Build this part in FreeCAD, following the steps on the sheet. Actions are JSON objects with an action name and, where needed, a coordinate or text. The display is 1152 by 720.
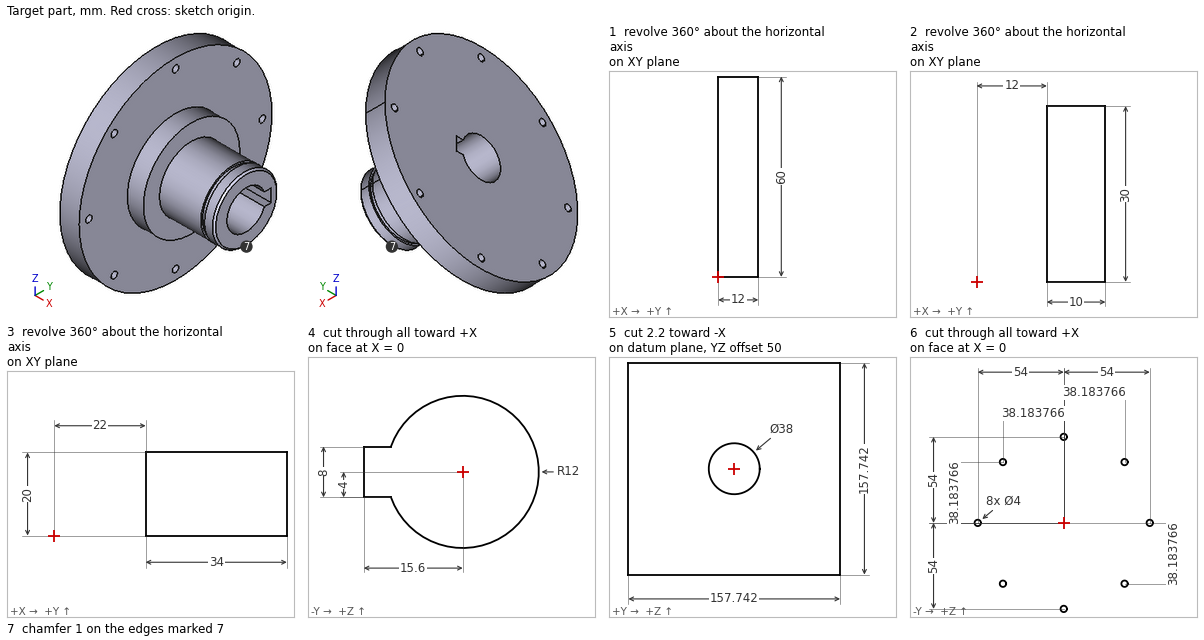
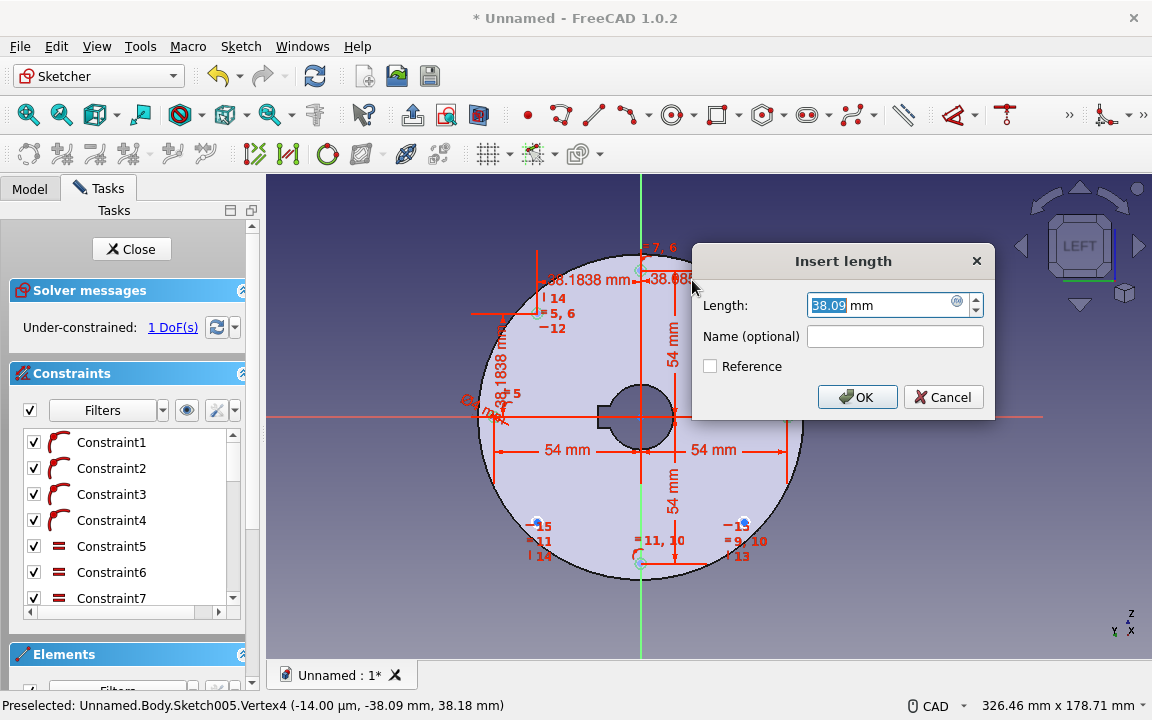
{"action": "type", "text": "38.183766"}
{"action": "key", "text": "Return"}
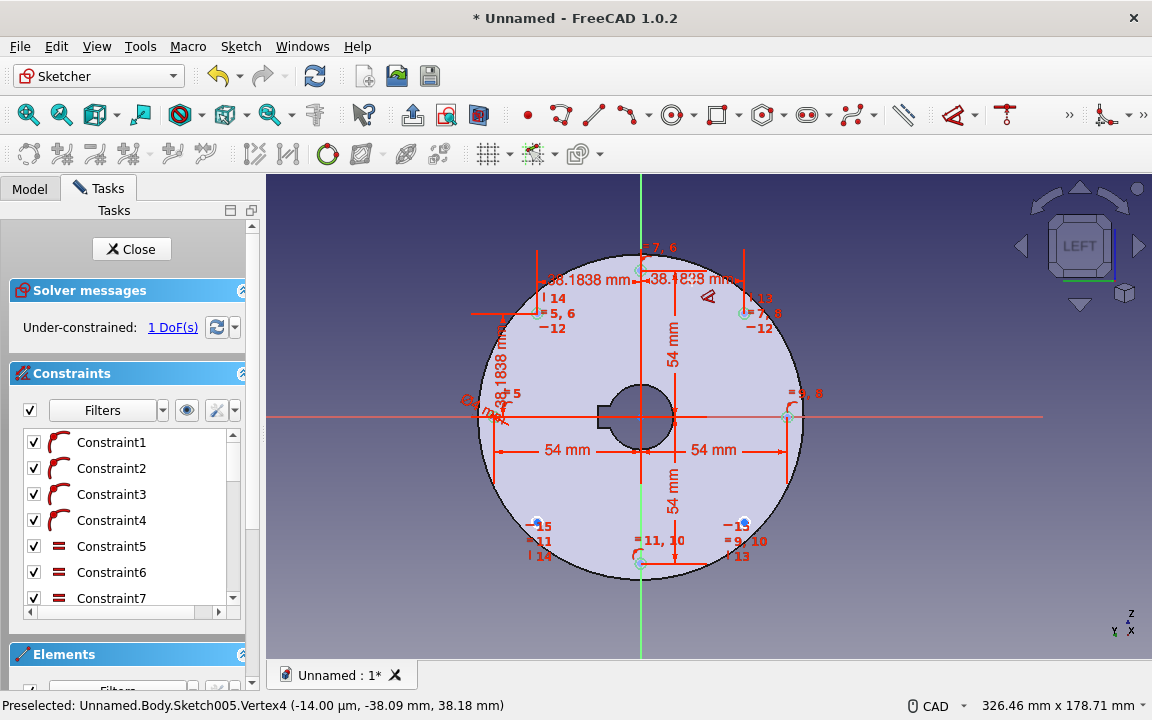
{"action": "left_click", "coordinate": [744, 522]}
{"action": "left_click", "coordinate": [778, 494]}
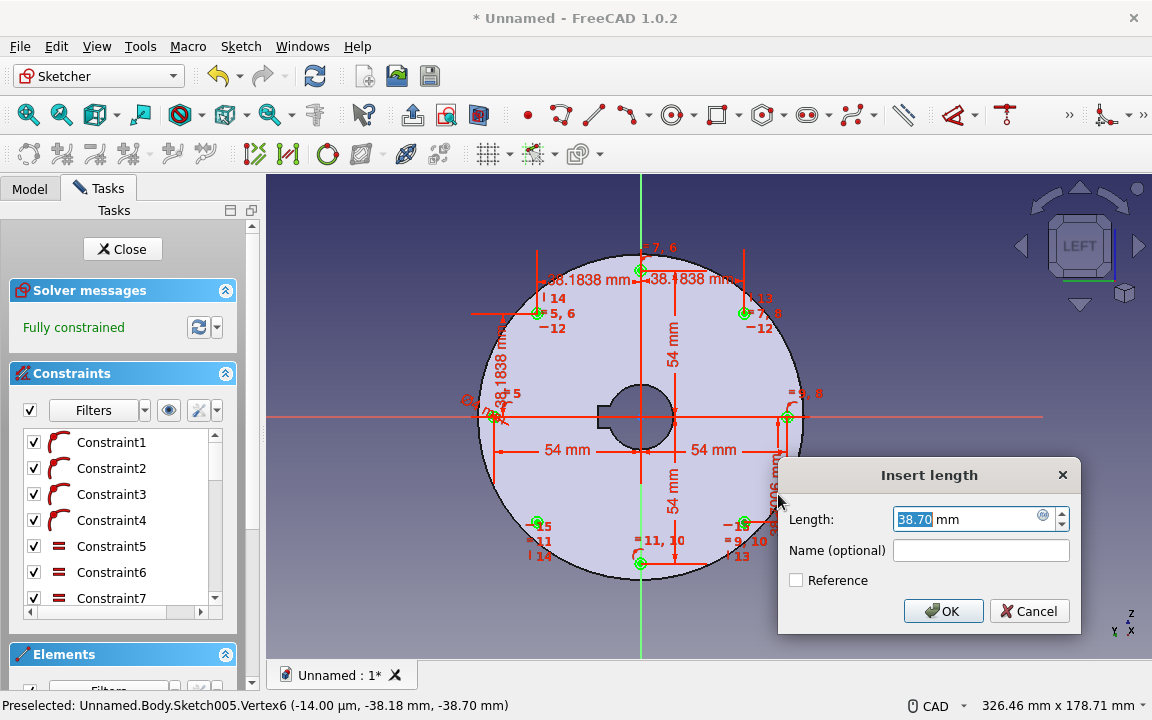
{"action": "type", "text": "38.183766"}
{"action": "key", "text": "Return"}
{"action": "key", "text": "Escape"}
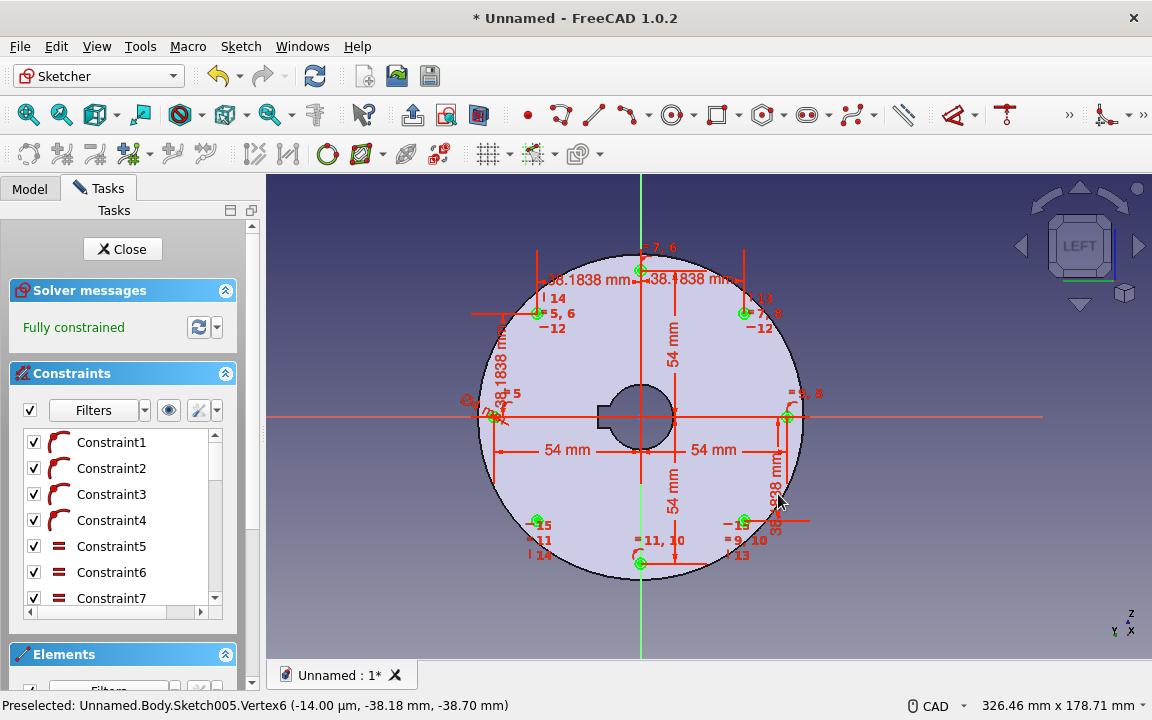
{"action": "left_click", "coordinate": [123, 249]}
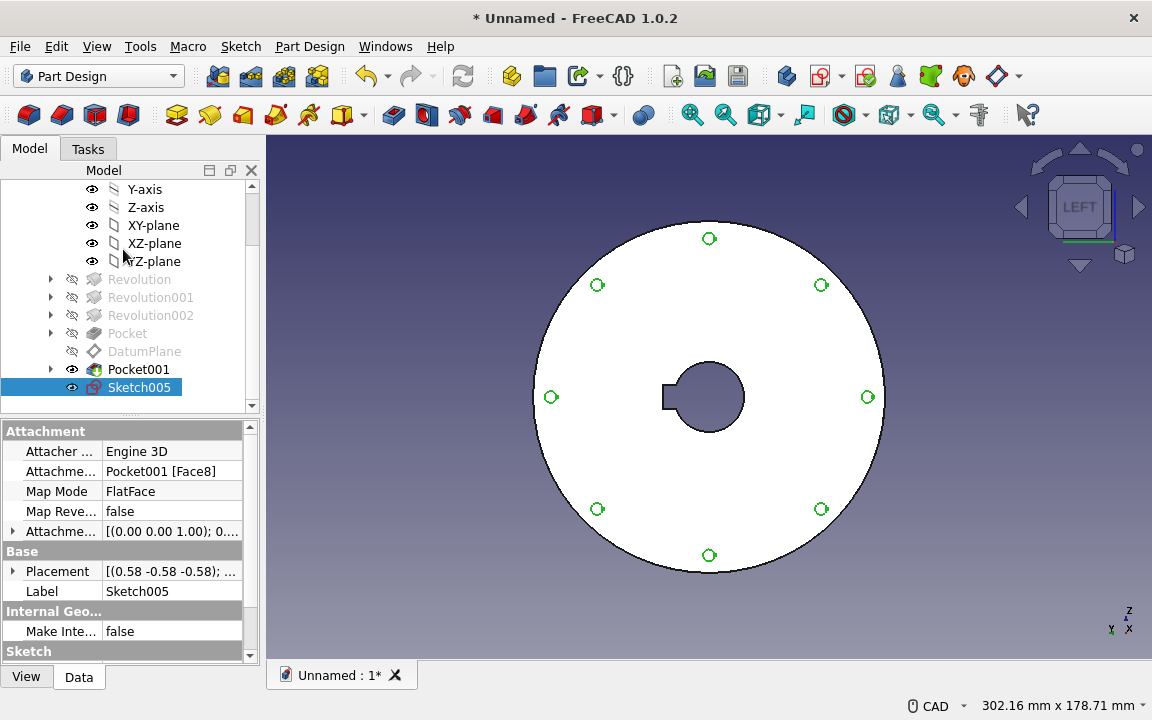
{"action": "left_click", "coordinate": [394, 116]}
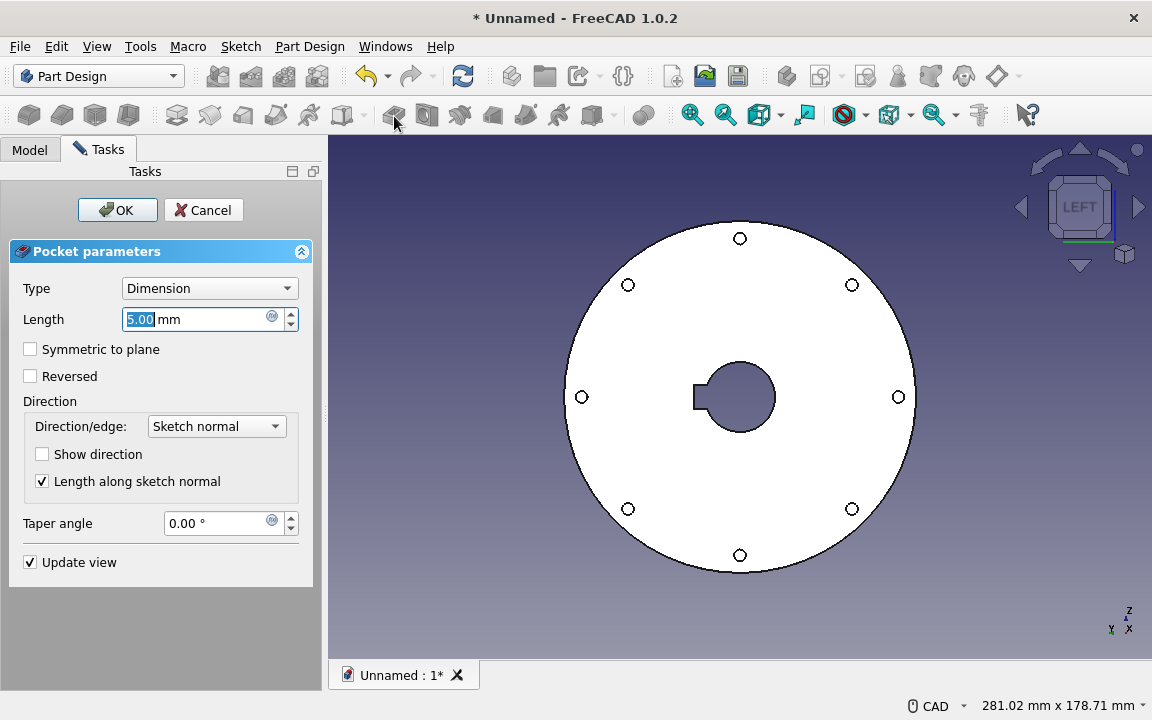
{"action": "left_click", "coordinate": [210, 288]}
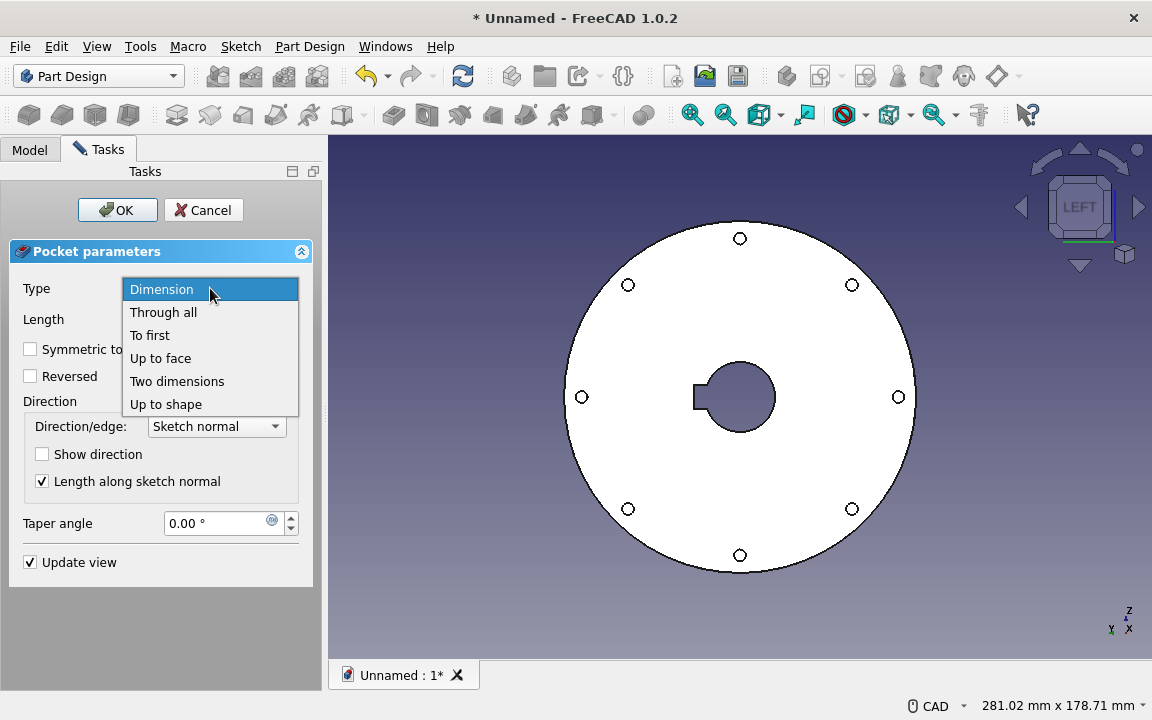
{"action": "left_click", "coordinate": [208, 312]}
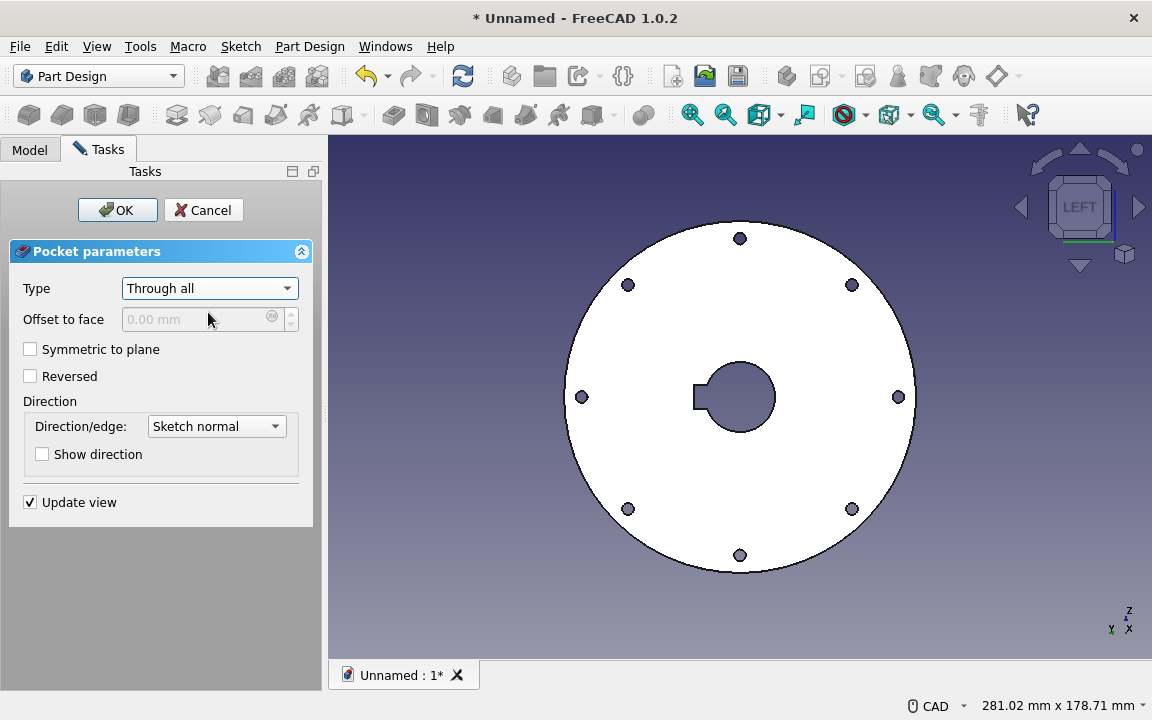
{"action": "left_click", "coordinate": [118, 210]}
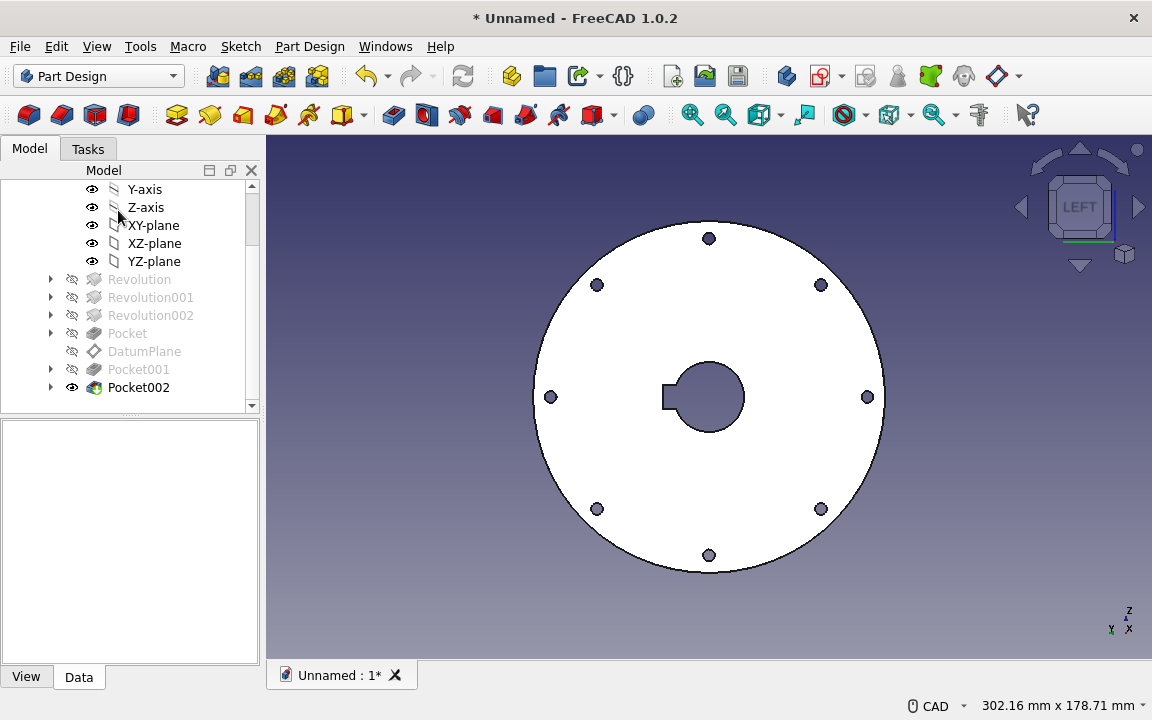
{"action": "key", "text": "0"}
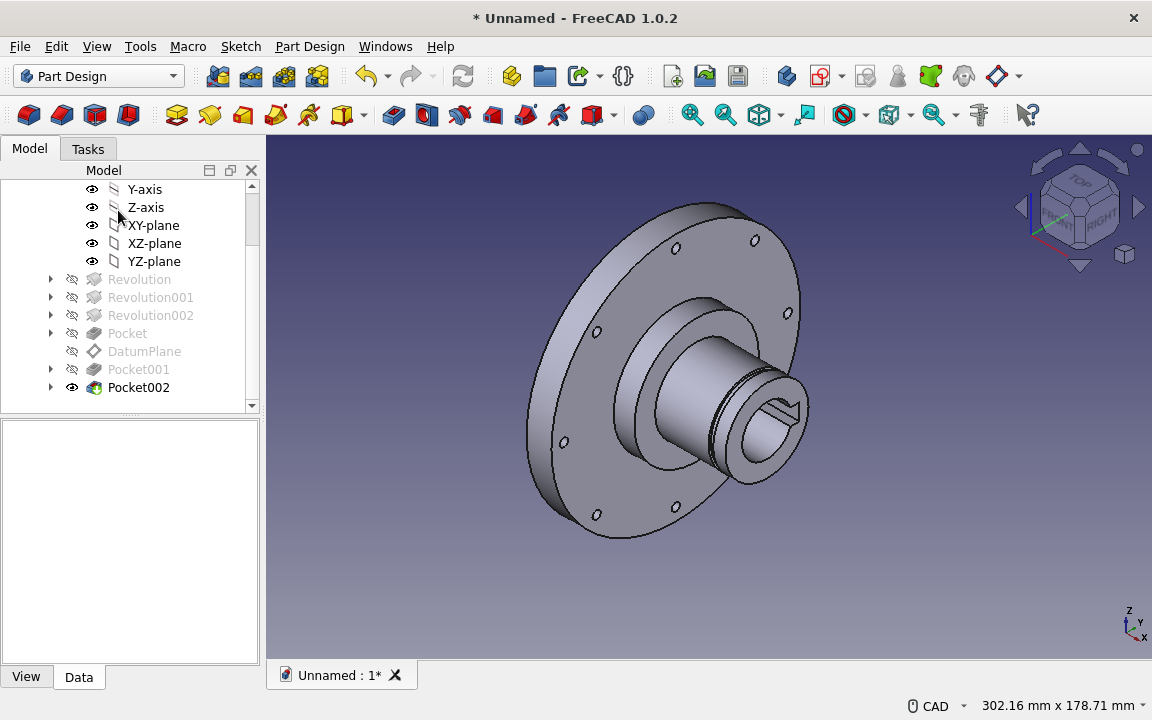
{"action": "left_click", "coordinate": [726, 453]}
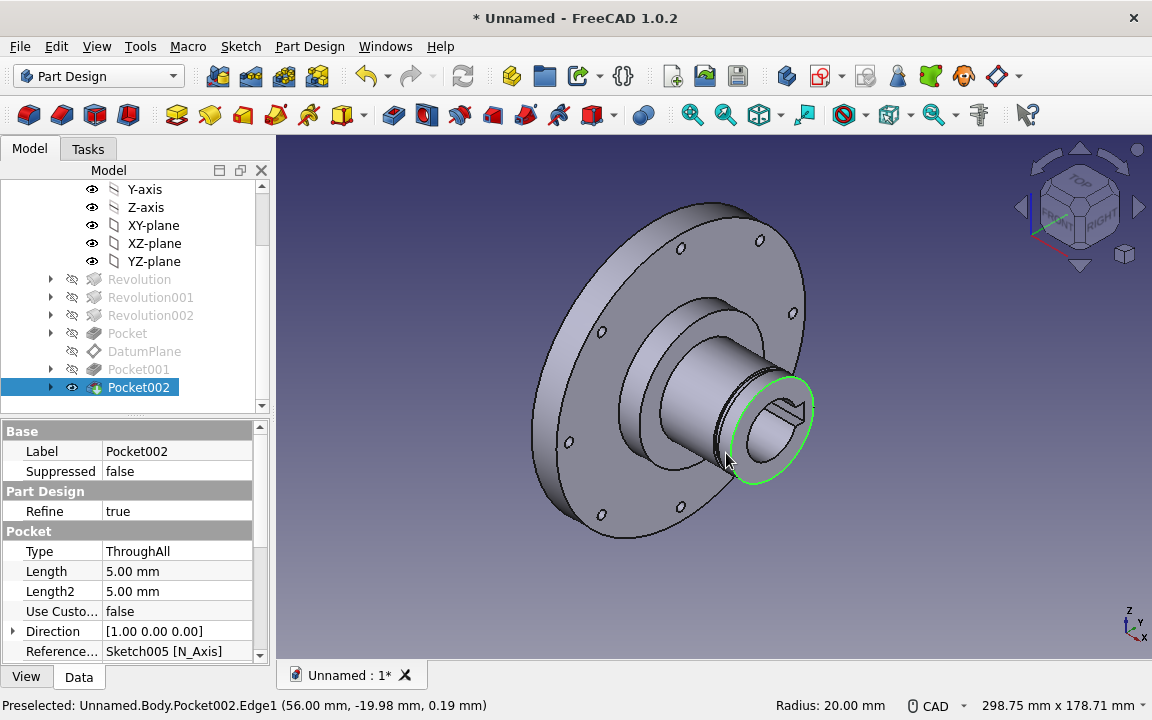
{"action": "left_click", "coordinate": [62, 116]}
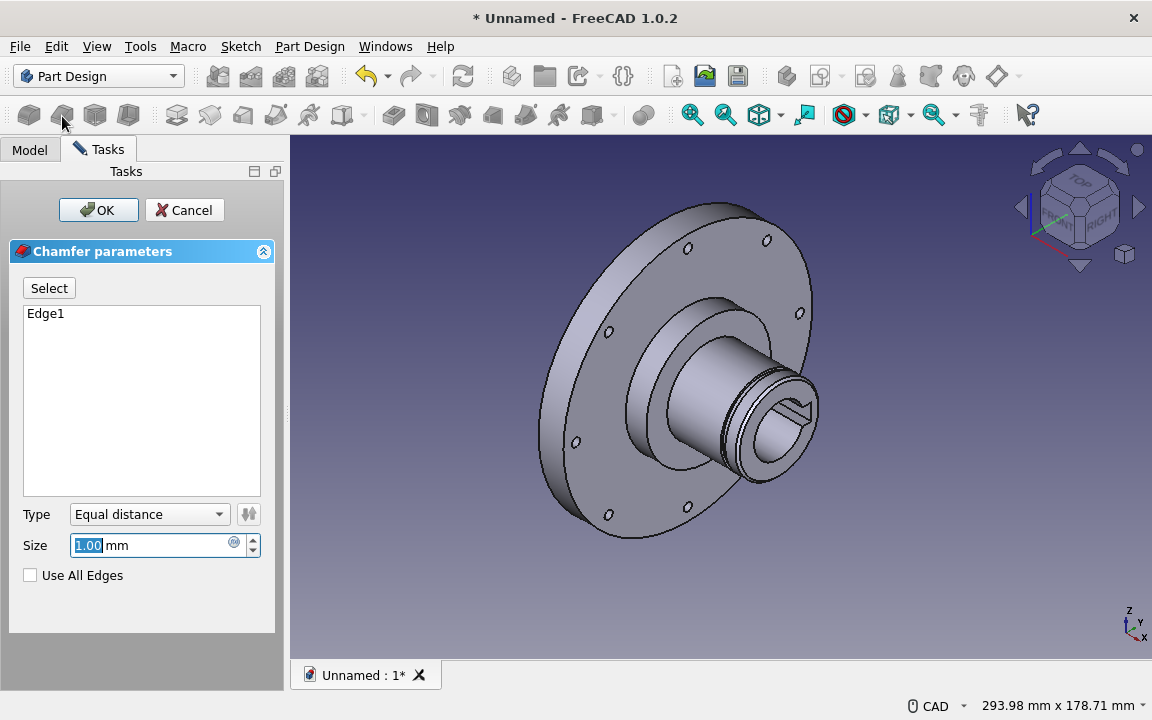
{"action": "type", "text": "1"}
{"action": "key", "text": "Tab"}